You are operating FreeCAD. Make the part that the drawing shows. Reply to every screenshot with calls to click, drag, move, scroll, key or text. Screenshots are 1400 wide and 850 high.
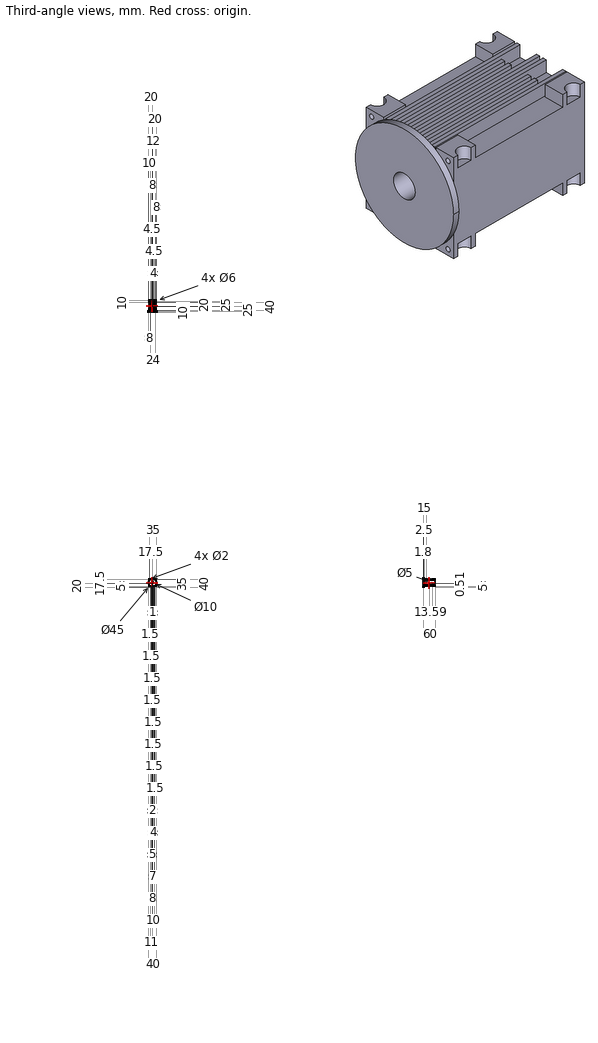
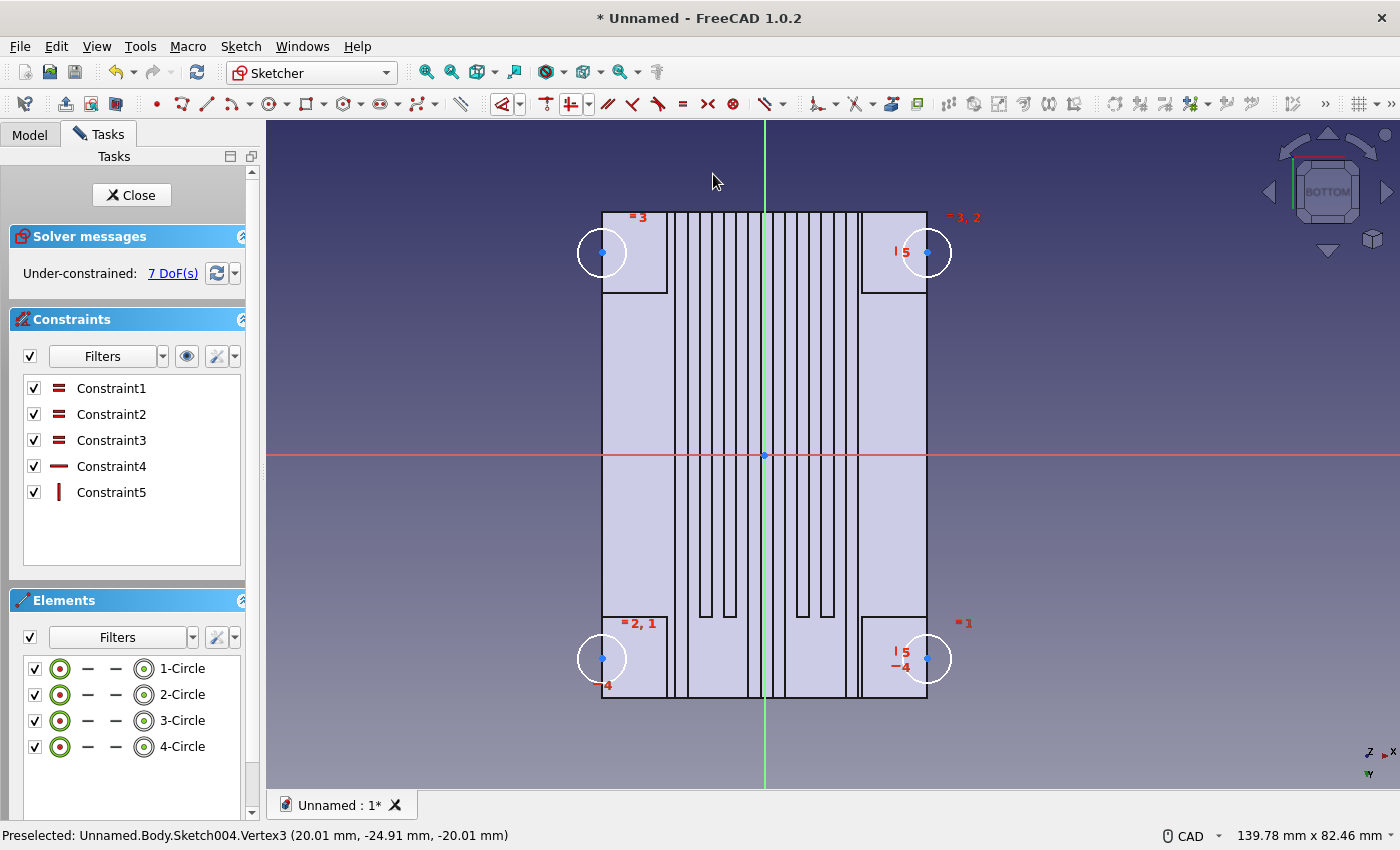
click(602, 659)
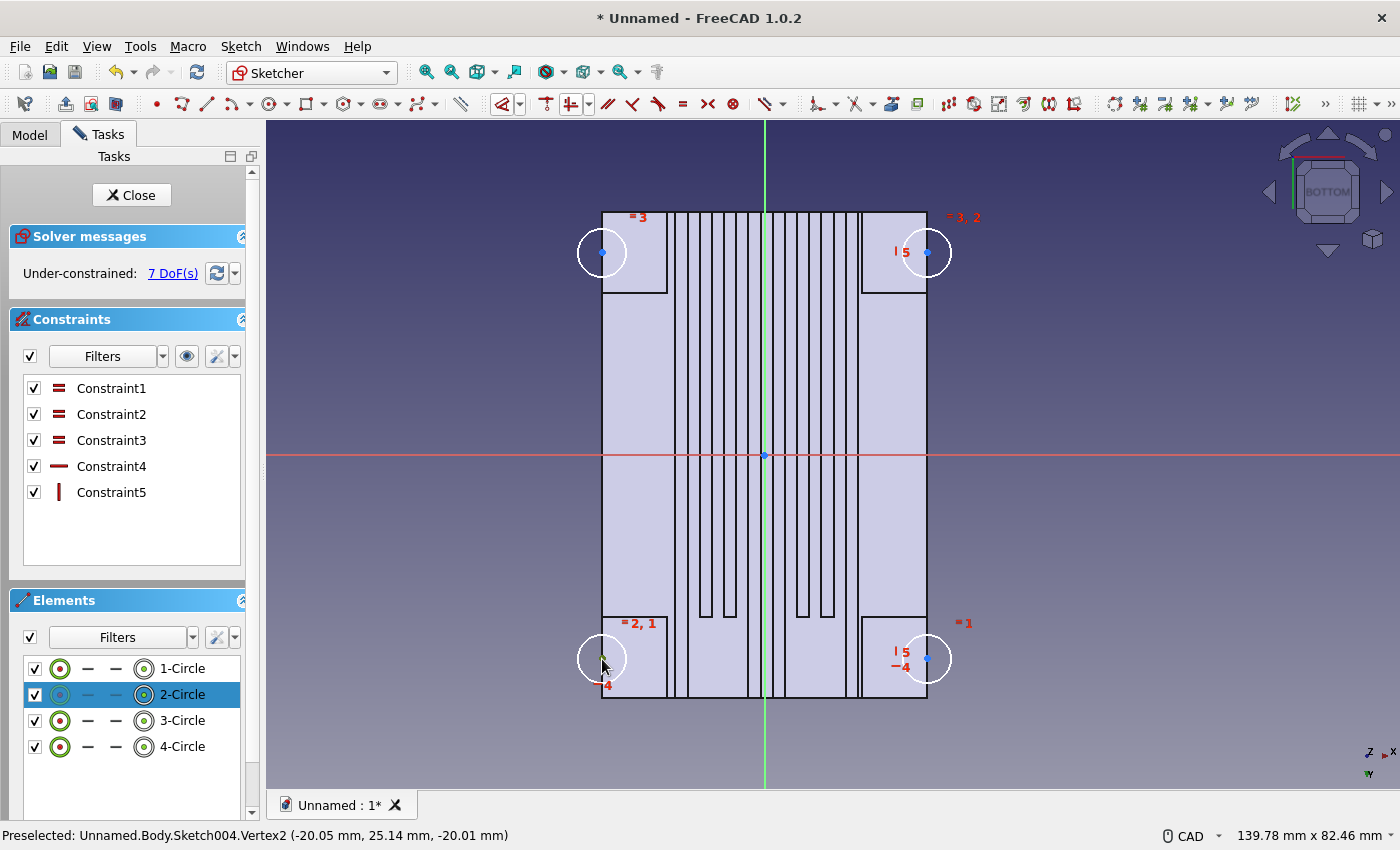
click(602, 253)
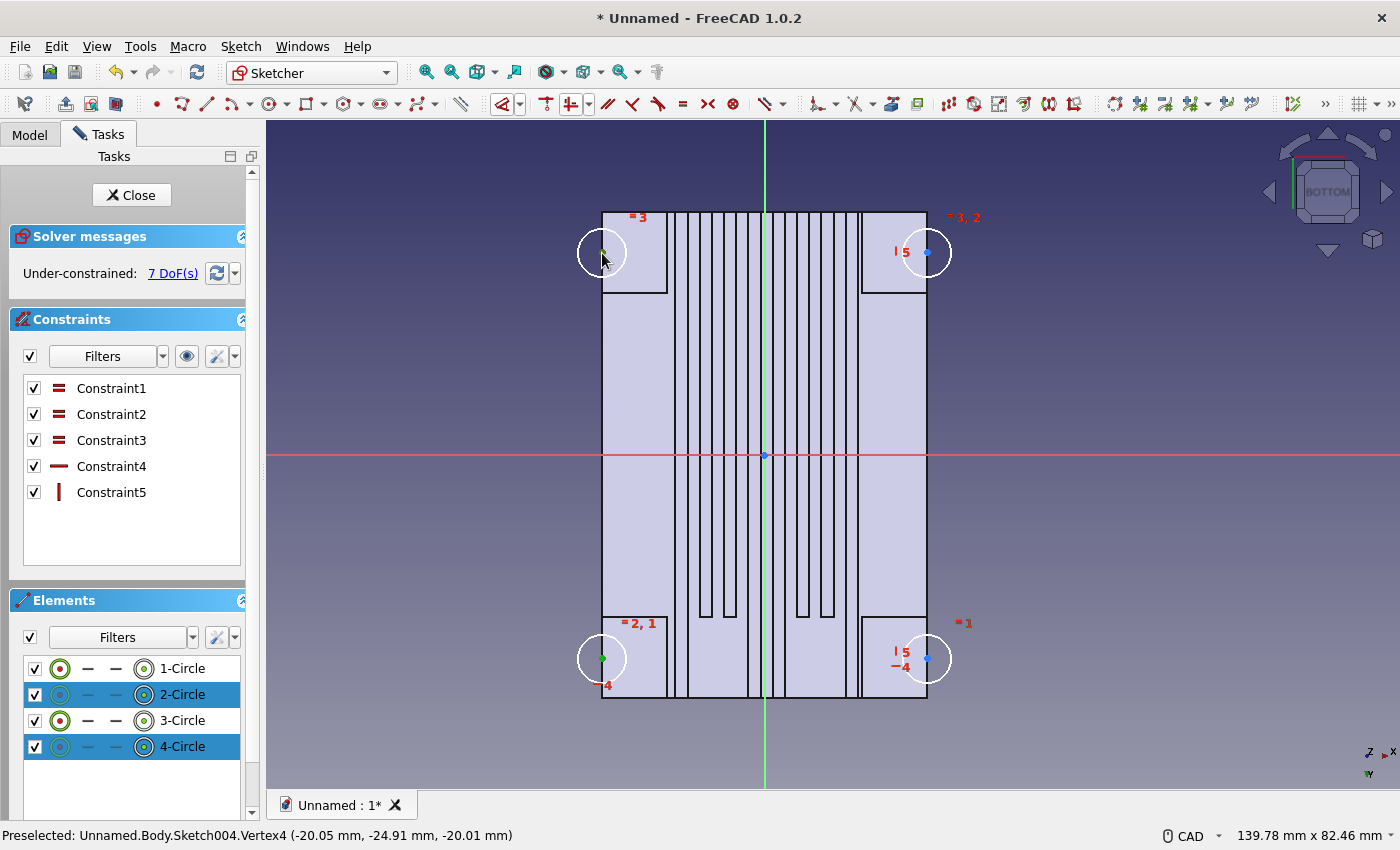
key(v)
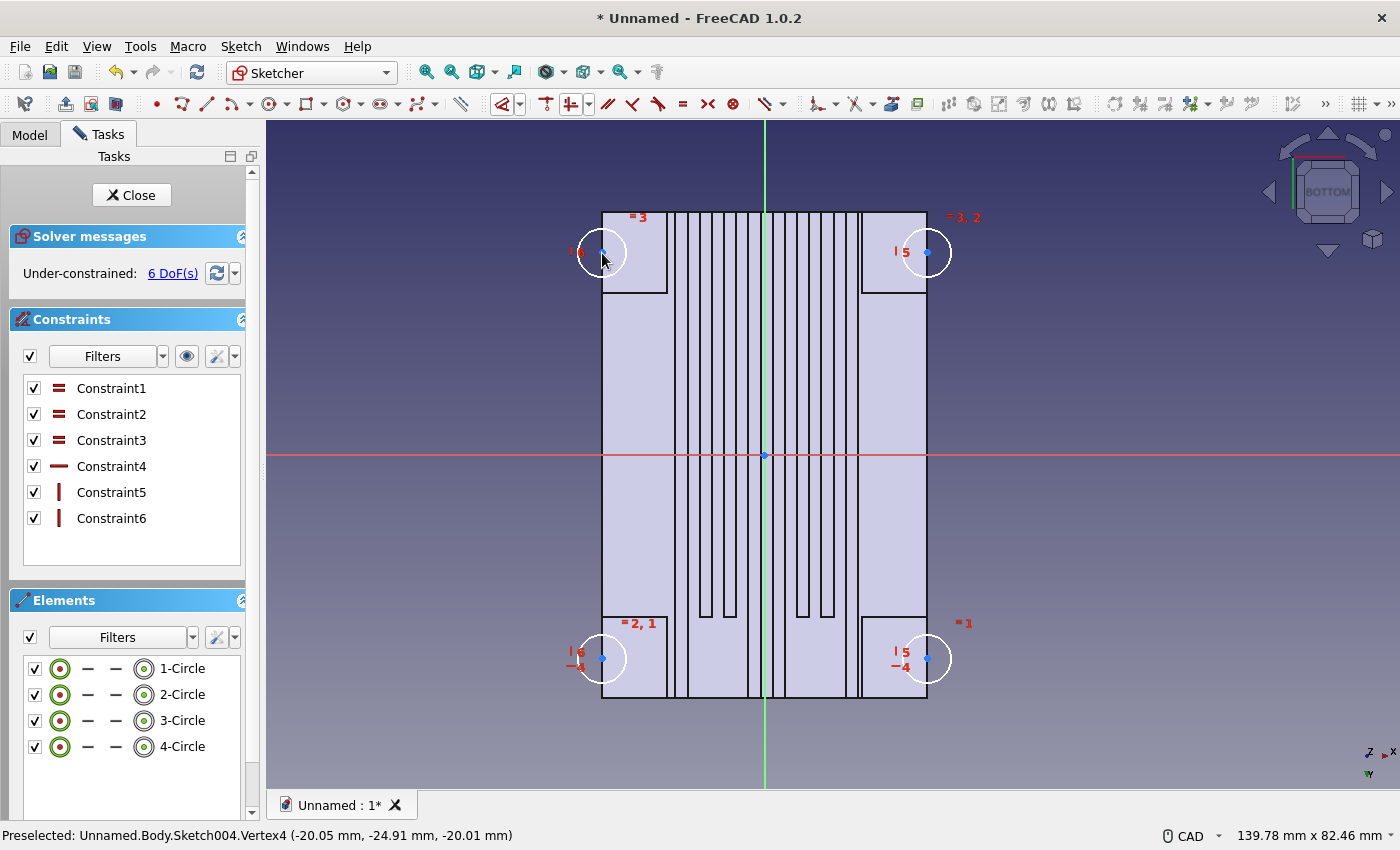
click(927, 253)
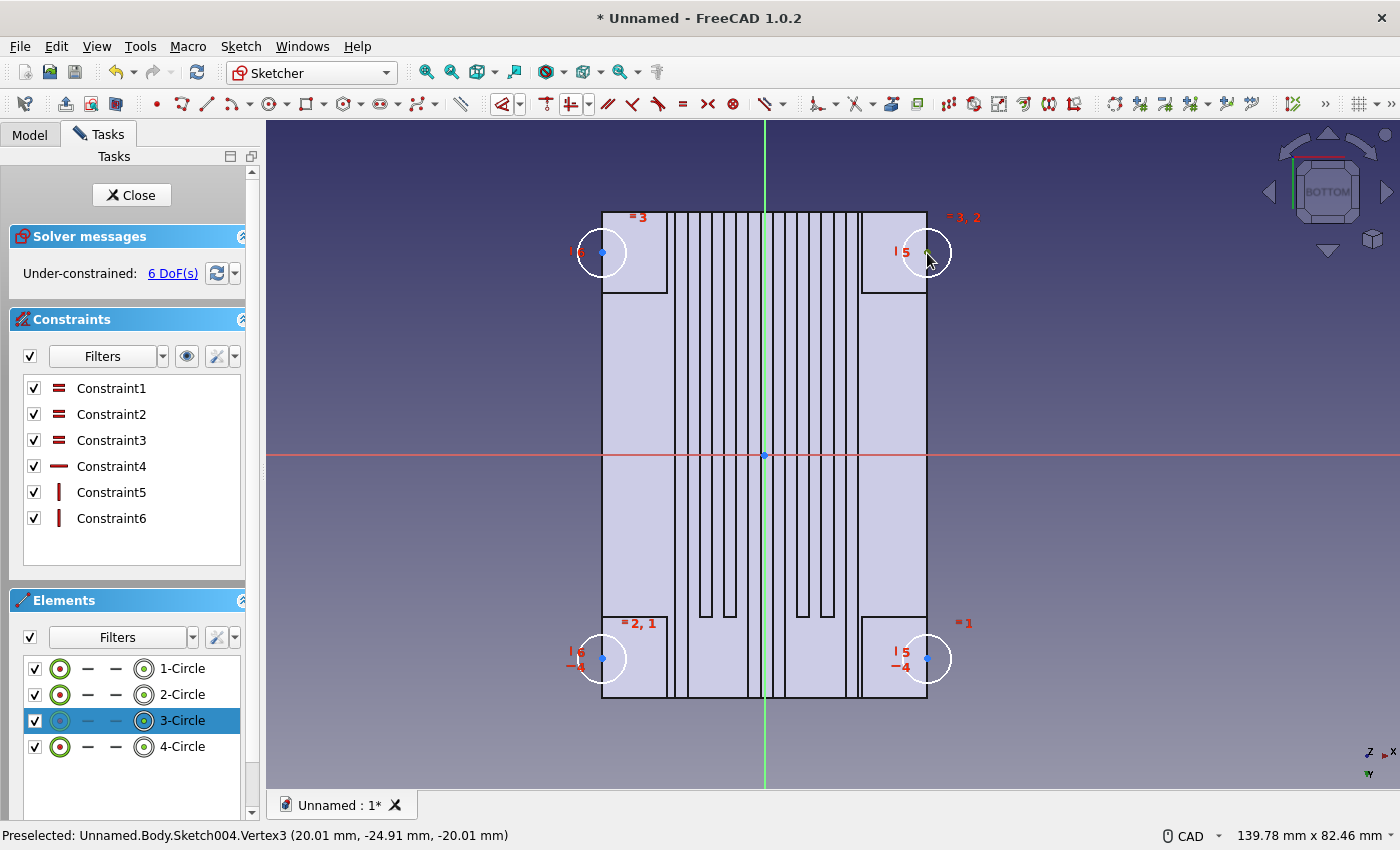
click(602, 253)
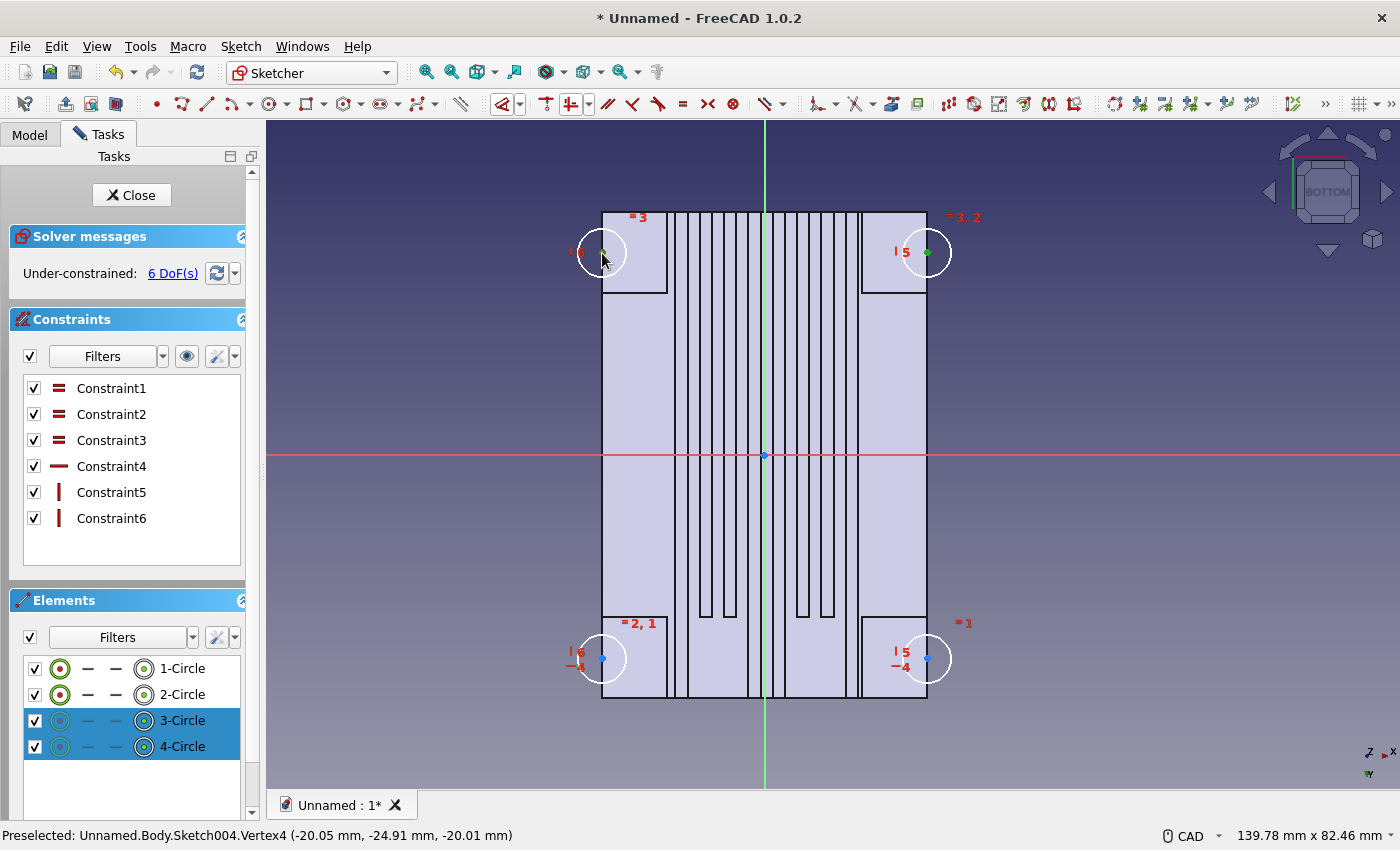
click(588, 104)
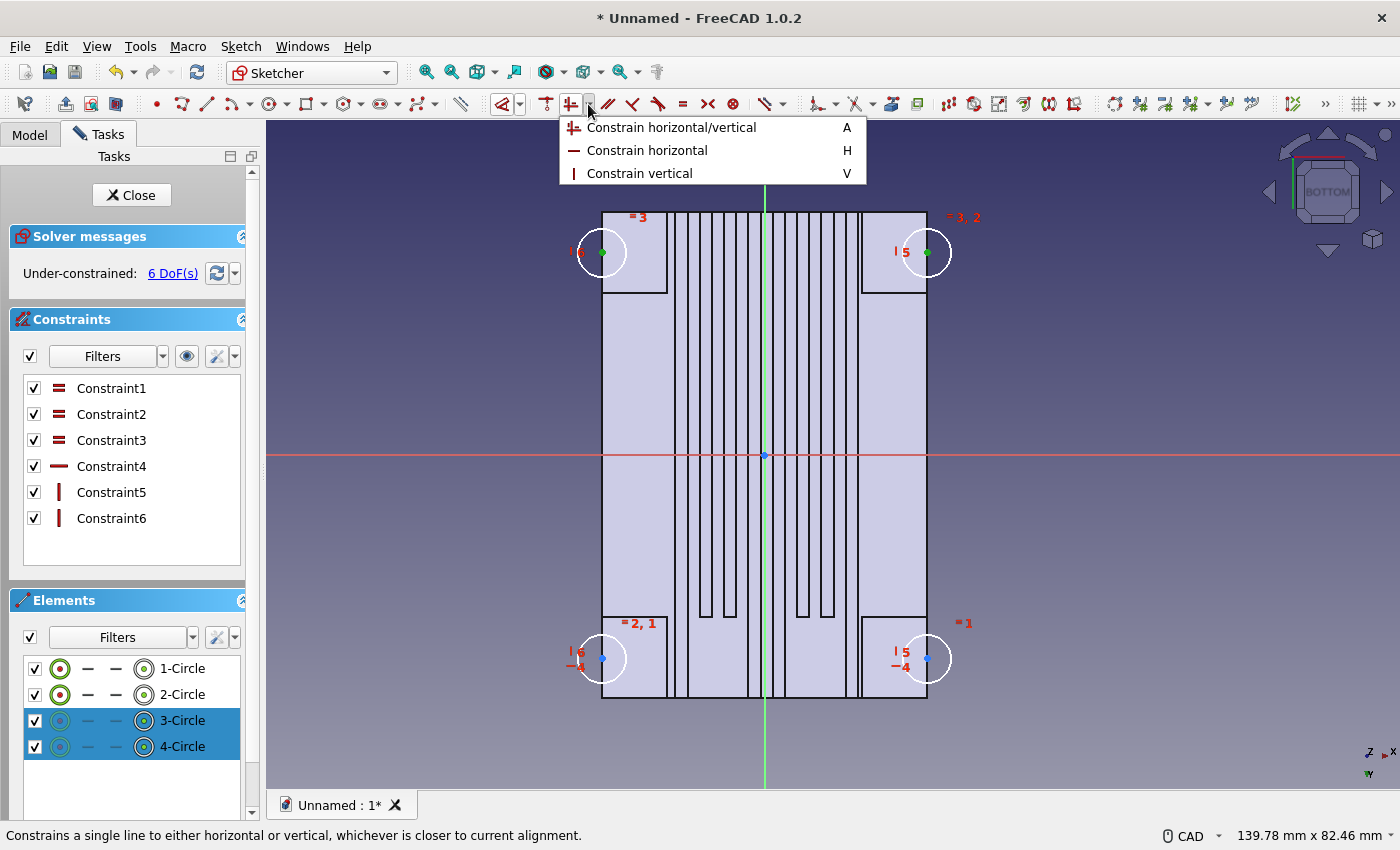
click(713, 150)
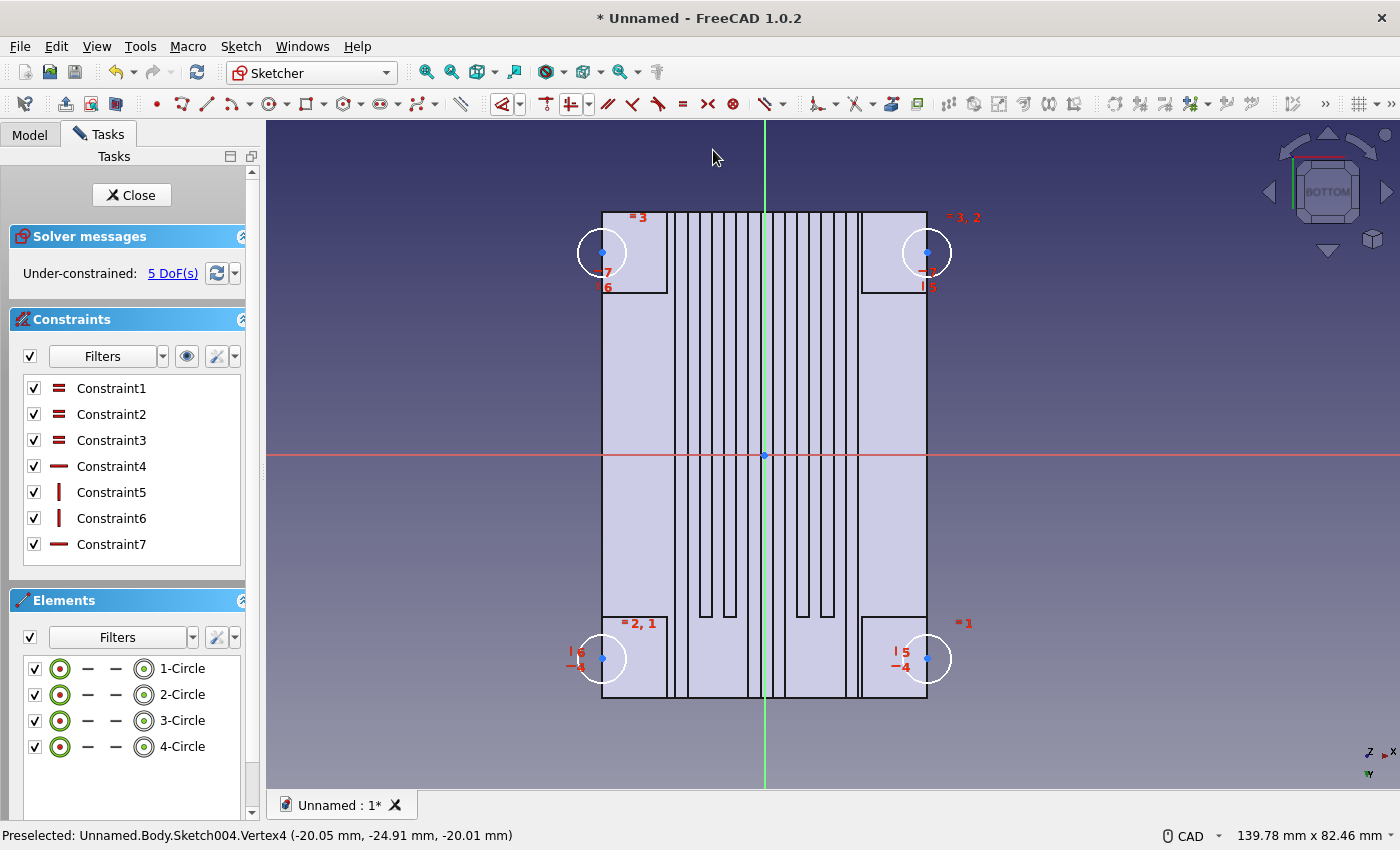
click(944, 642)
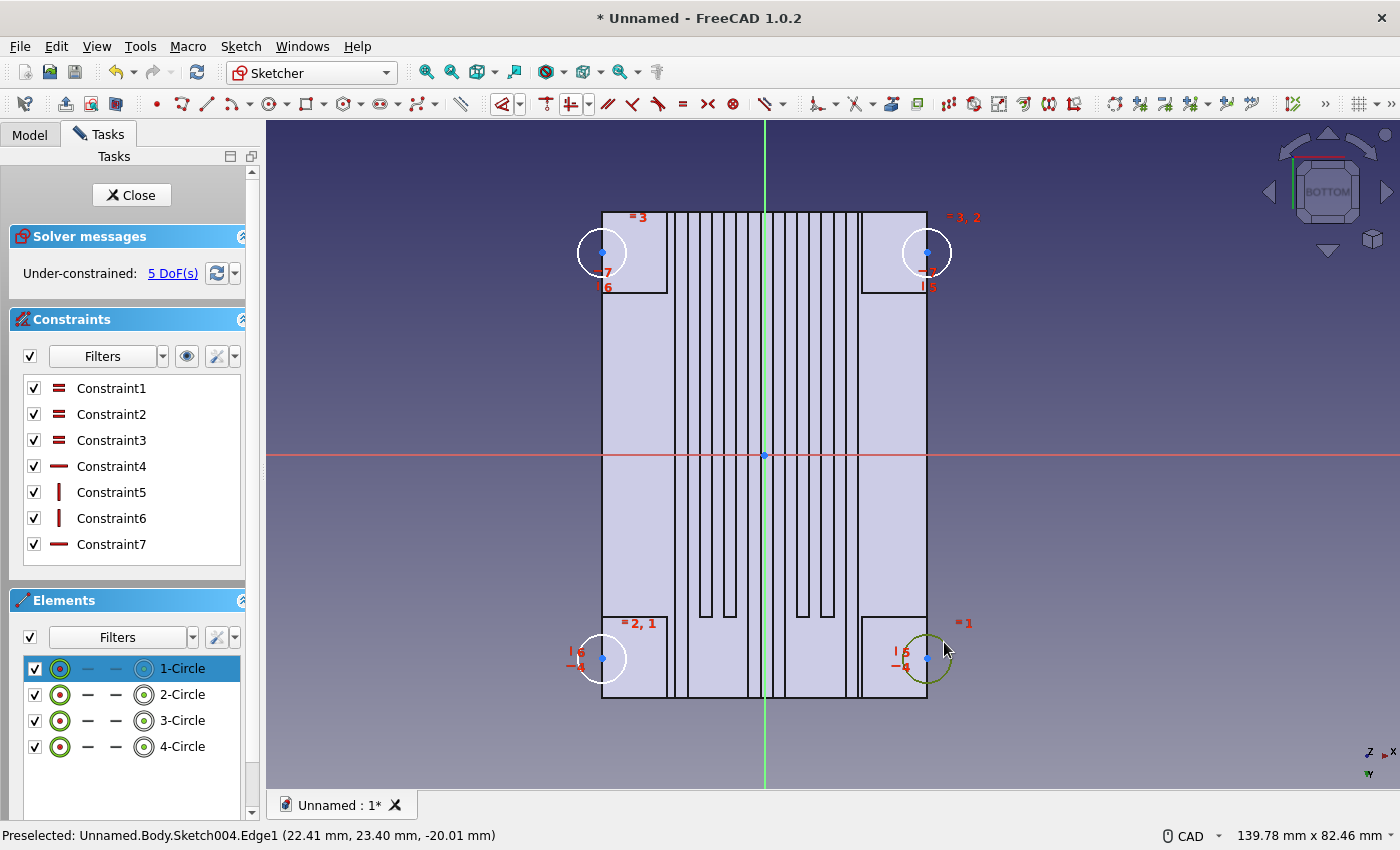
key(k)
key(o)